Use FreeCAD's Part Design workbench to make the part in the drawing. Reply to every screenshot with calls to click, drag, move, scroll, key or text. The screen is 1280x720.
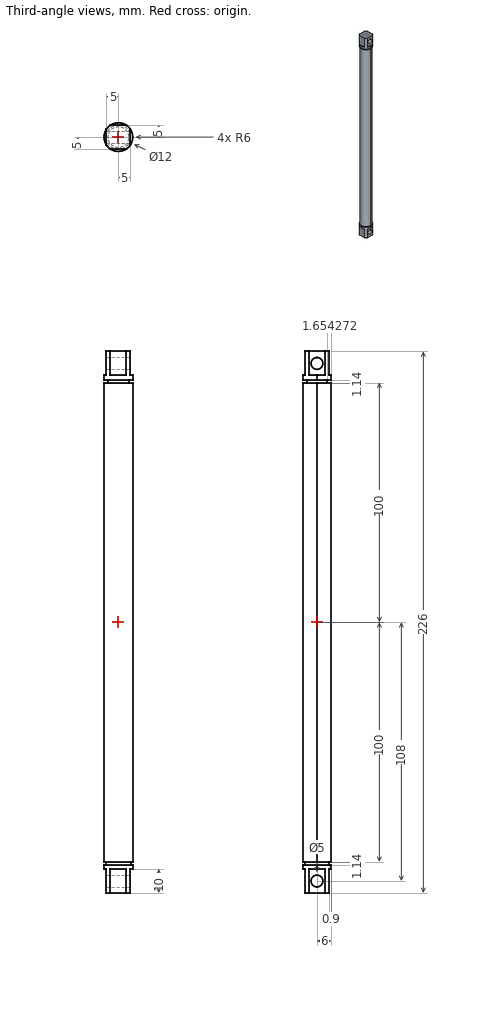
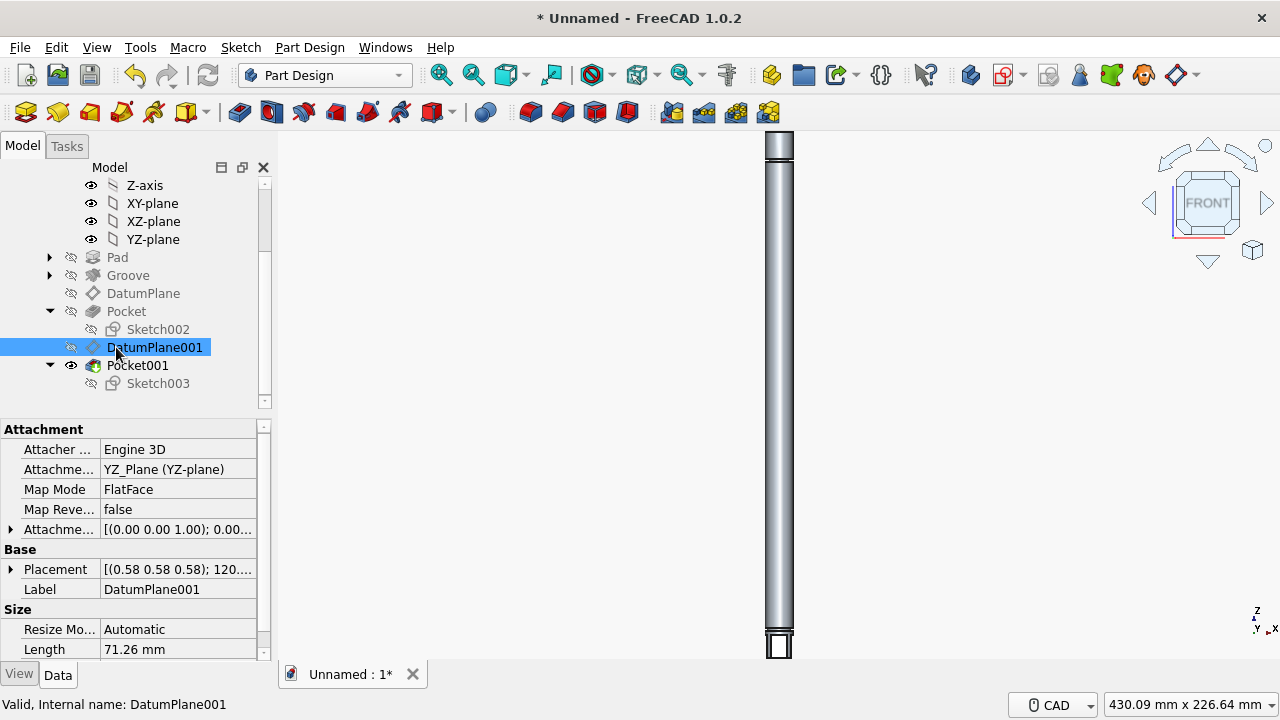
click(116, 311)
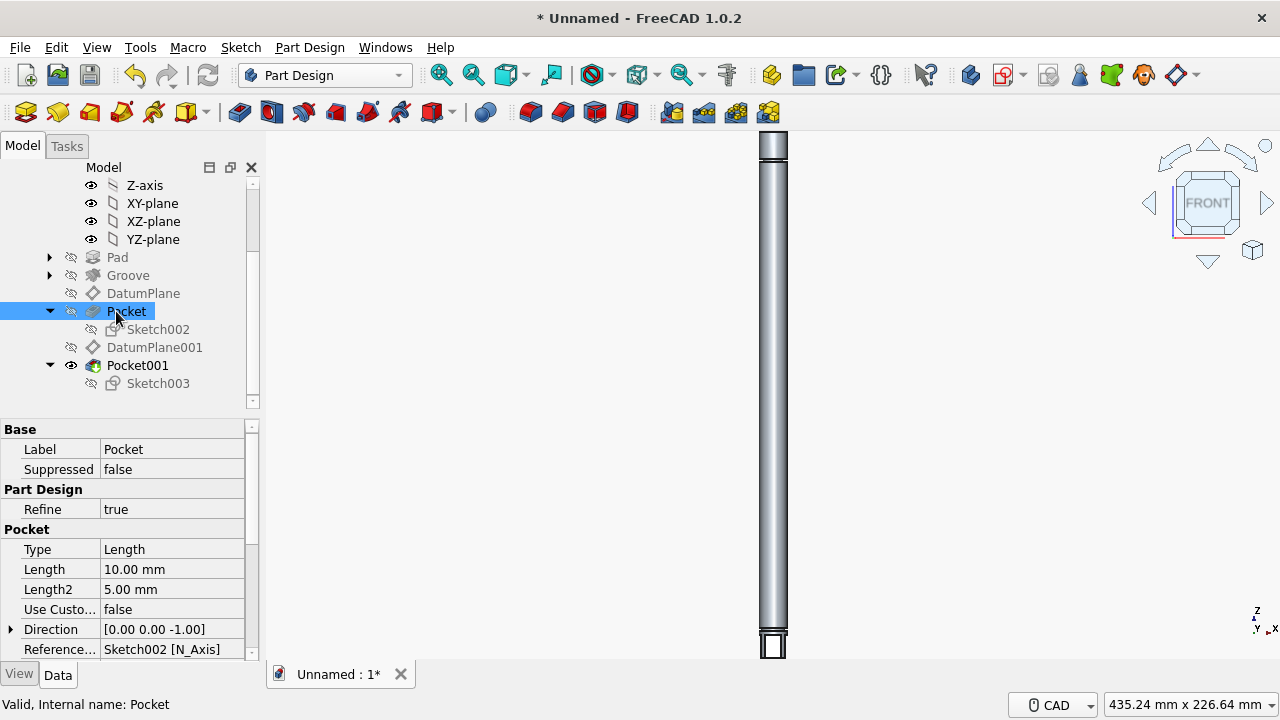
click(116, 365, ctrl)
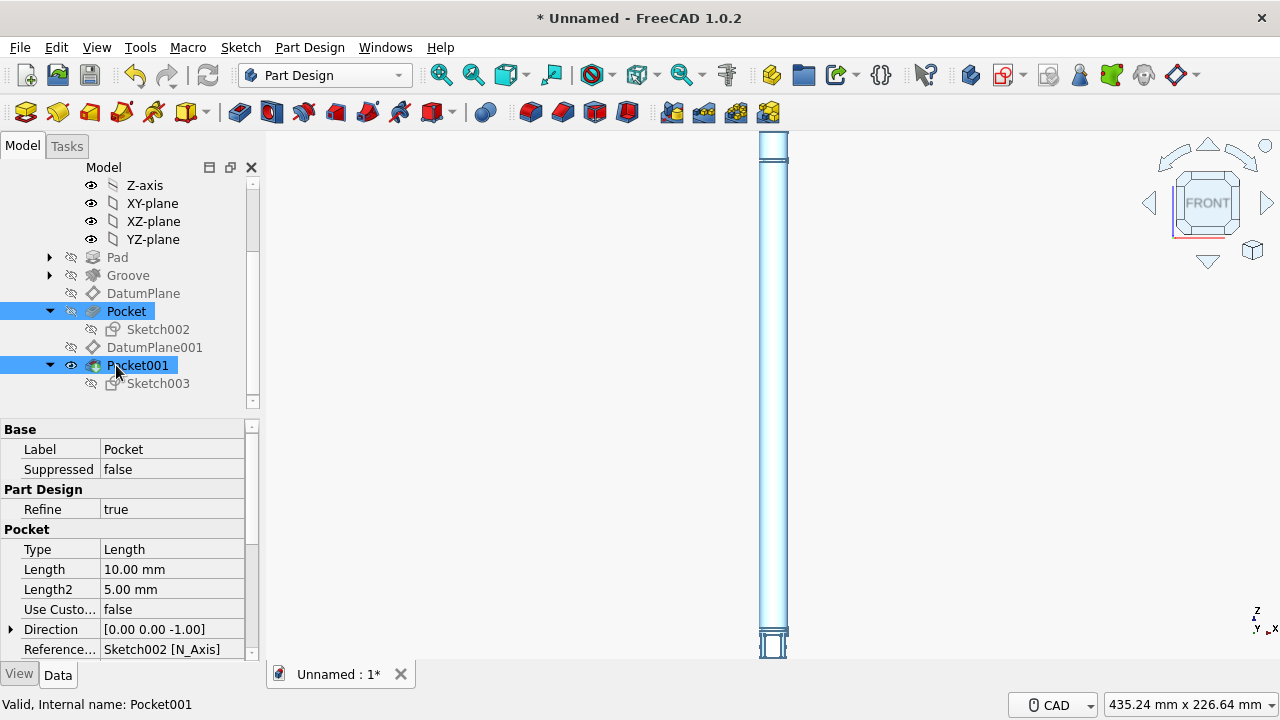
click(672, 112)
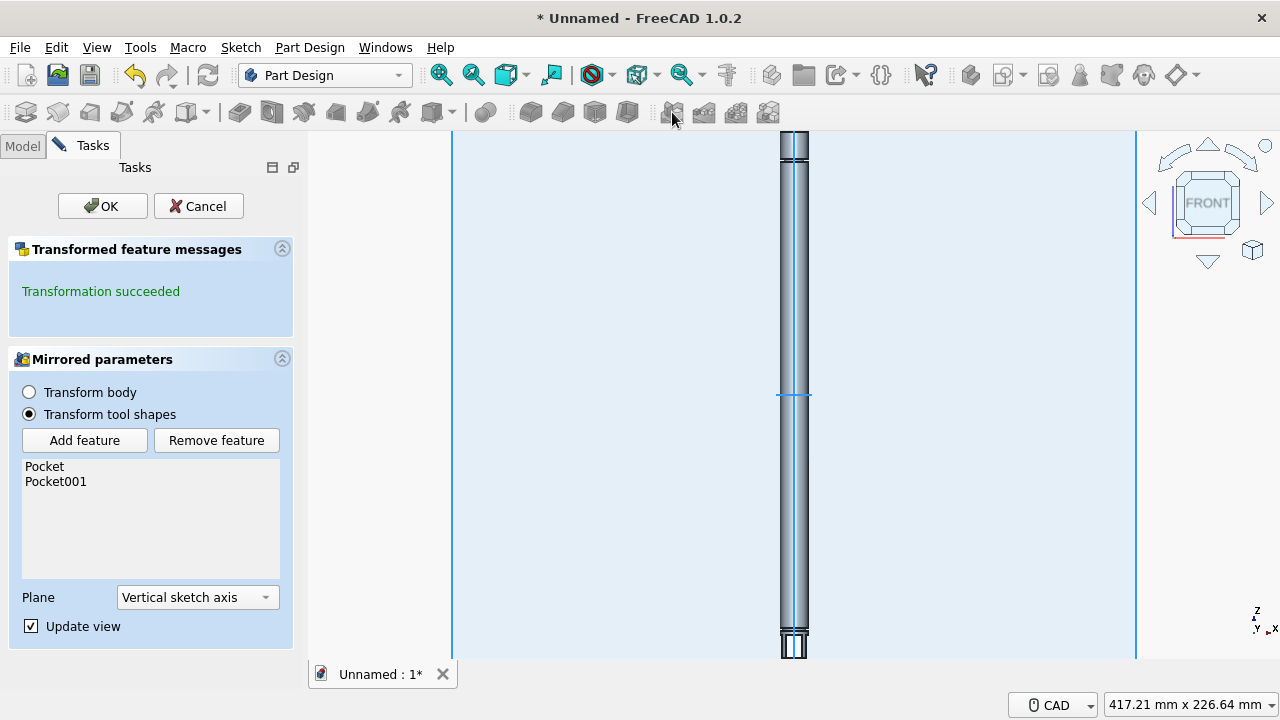
click(198, 598)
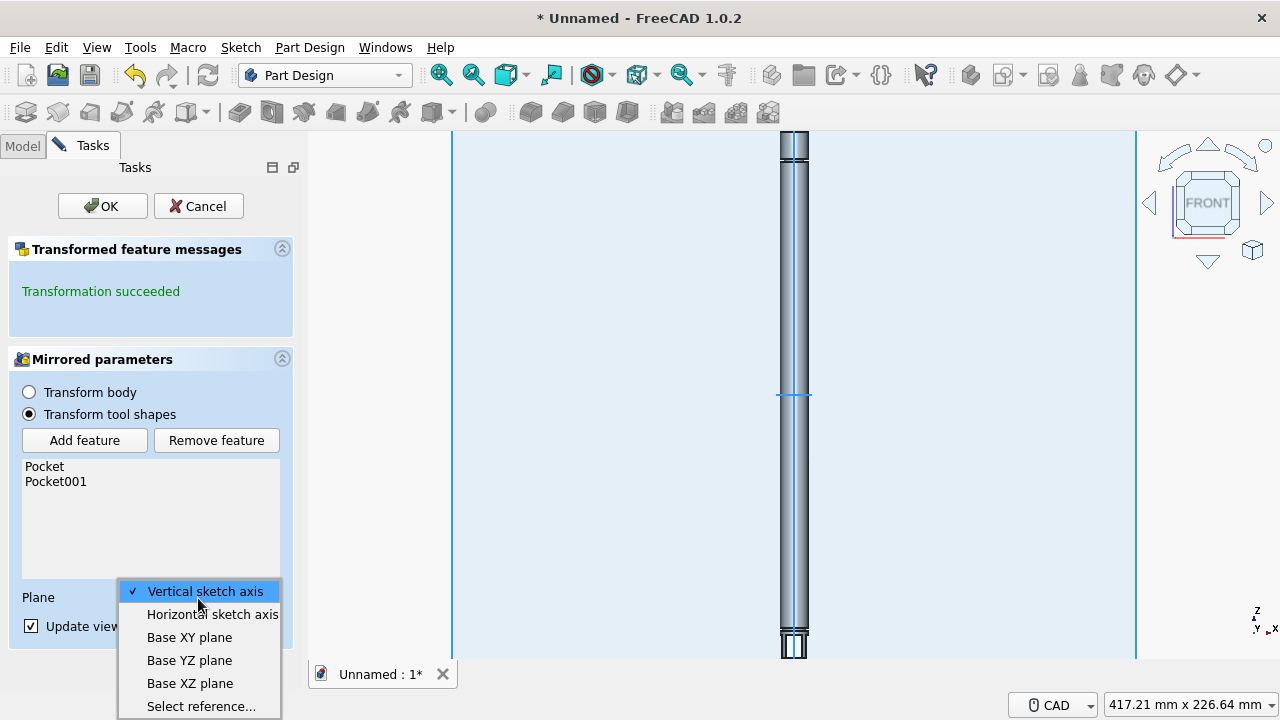
click(198, 638)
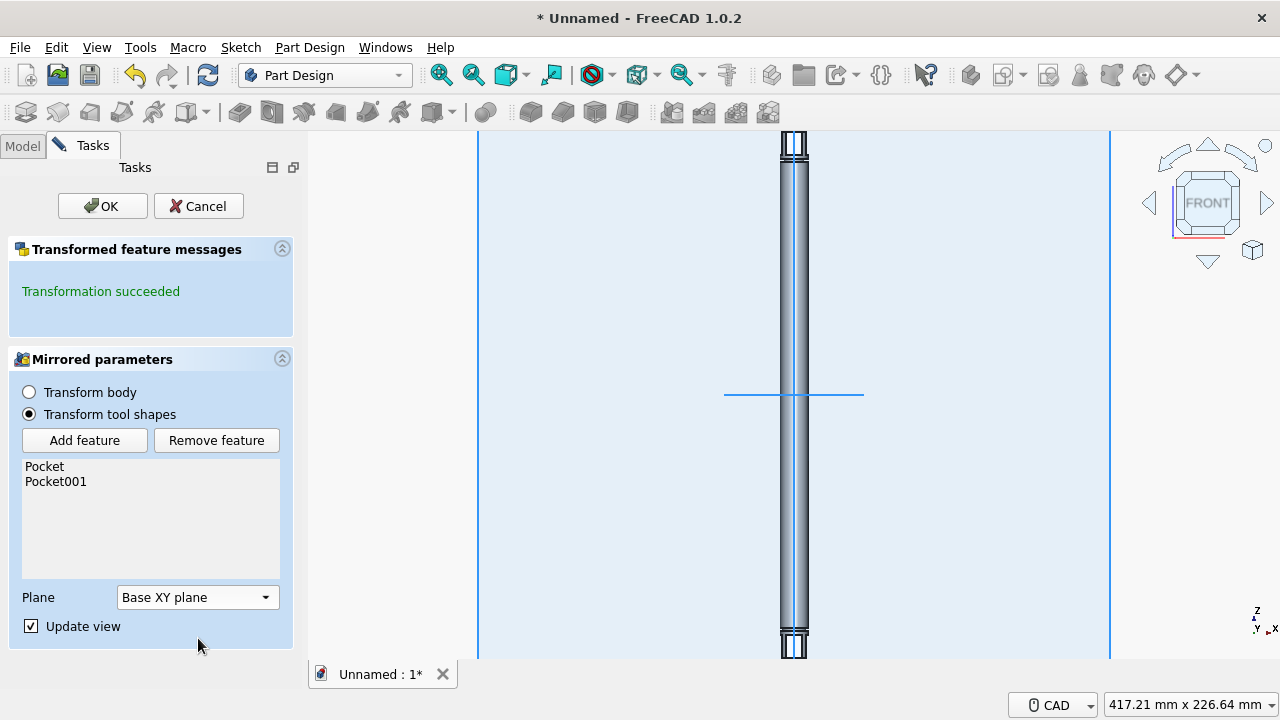
click(103, 206)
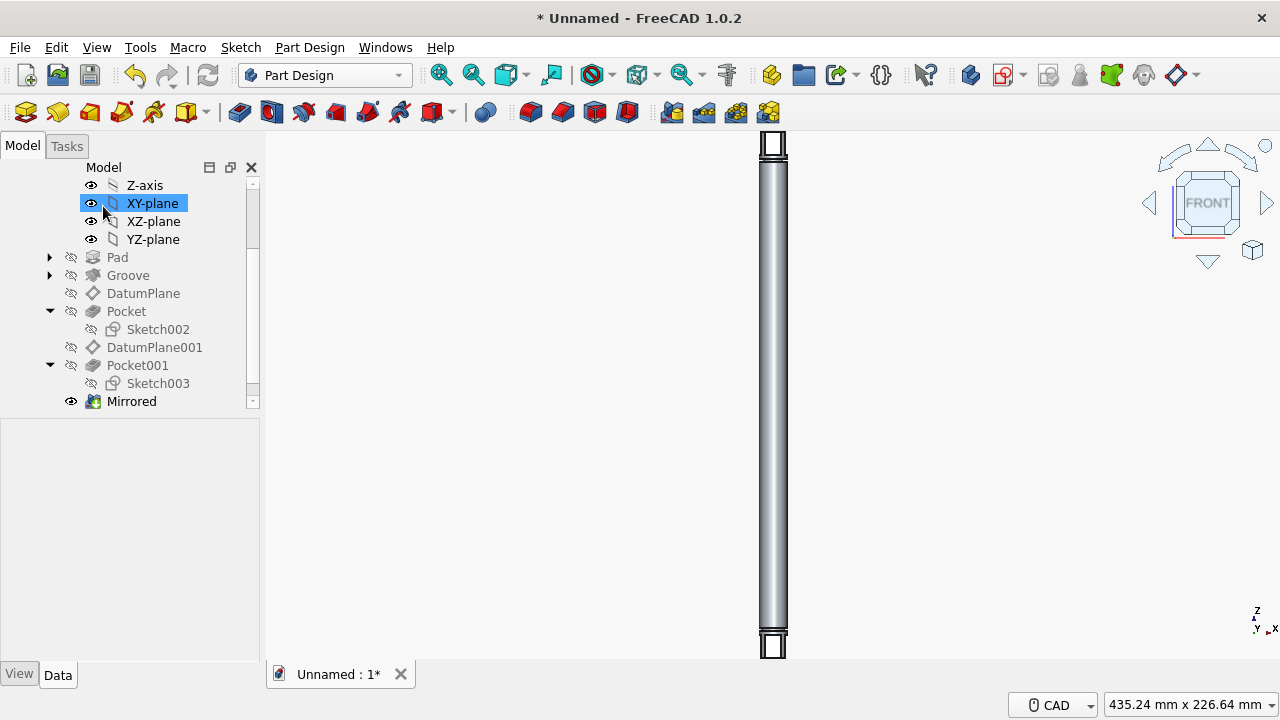
key(0)